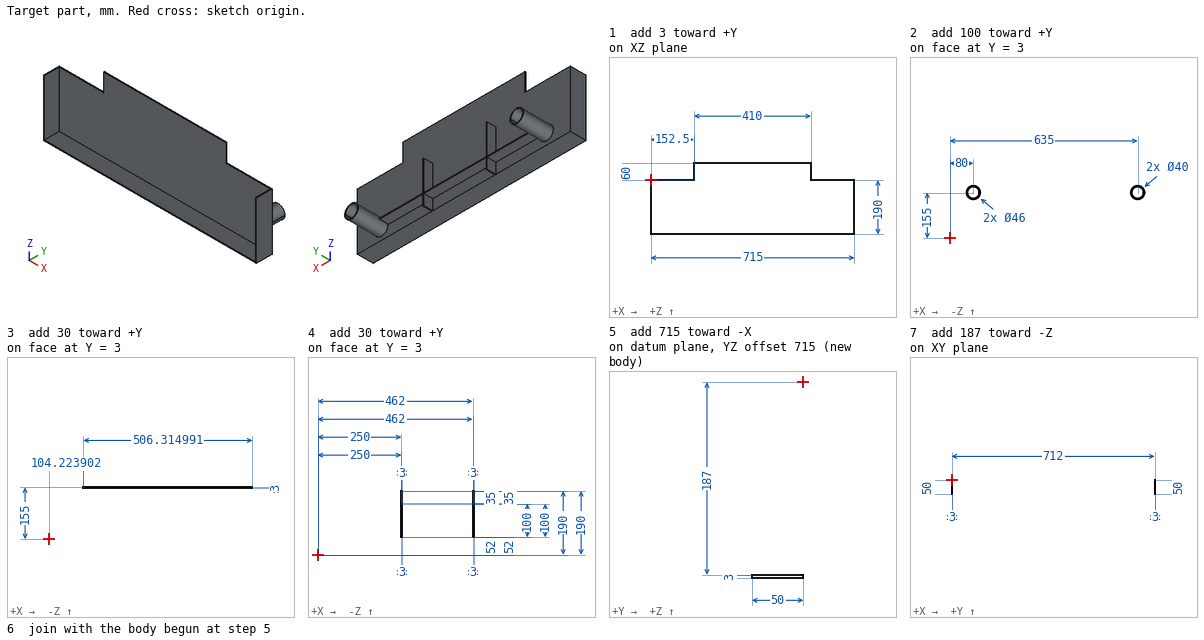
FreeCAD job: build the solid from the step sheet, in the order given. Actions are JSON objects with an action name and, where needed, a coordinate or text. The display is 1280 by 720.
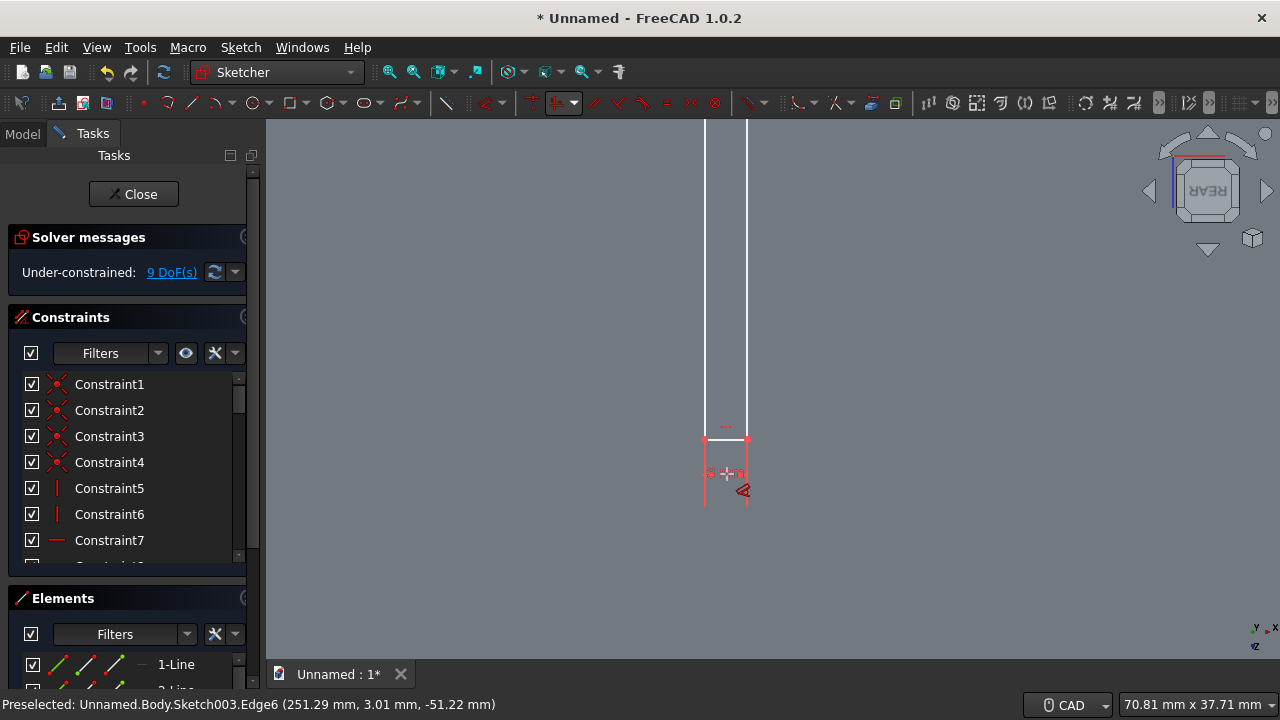
{"action": "scroll", "coordinate": [729, 446], "scroll_direction": "down", "scroll_amount": 12}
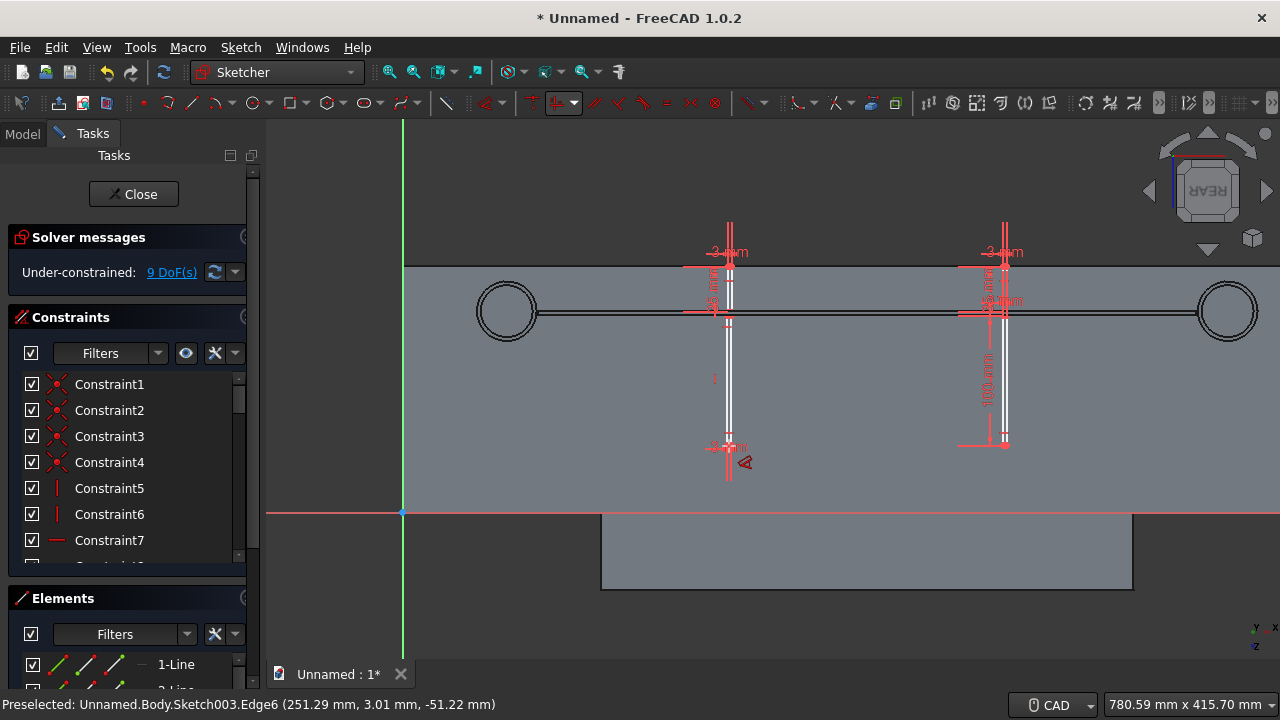
{"action": "scroll", "coordinate": [727, 420], "scroll_direction": "up", "scroll_amount": 7}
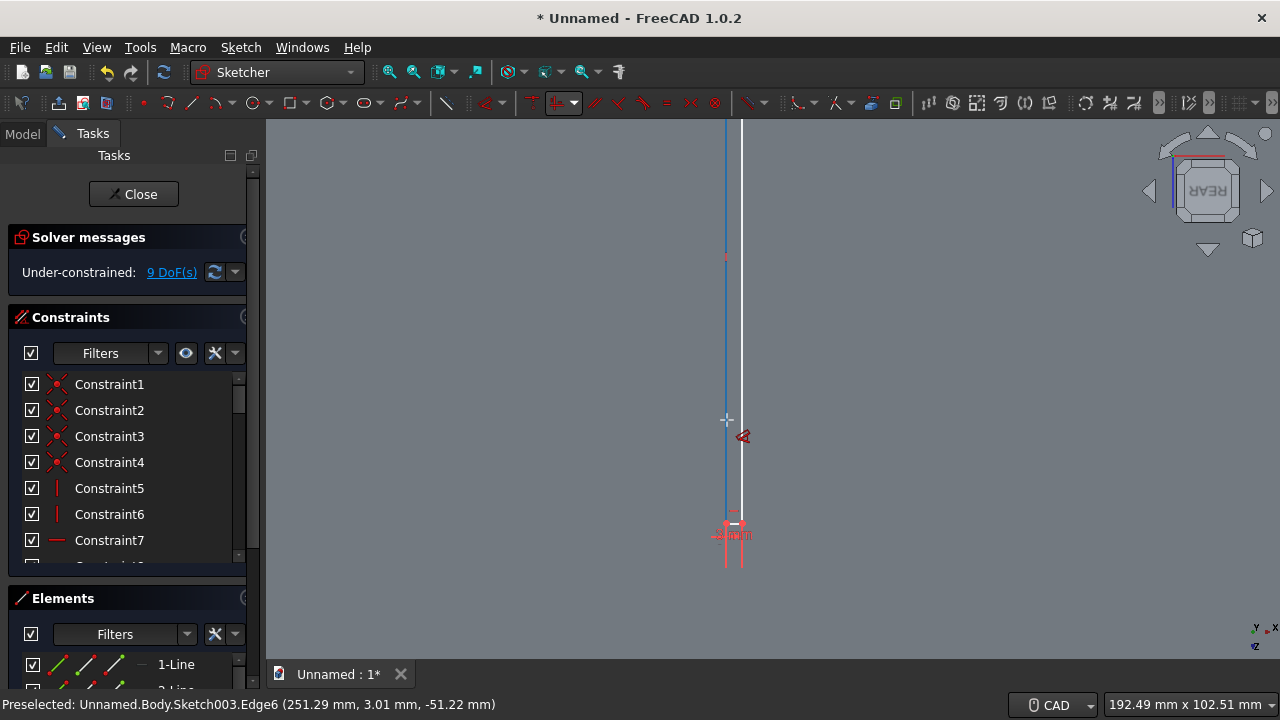
{"action": "left_click", "coordinate": [726, 418]}
{"action": "left_click", "coordinate": [760, 335]}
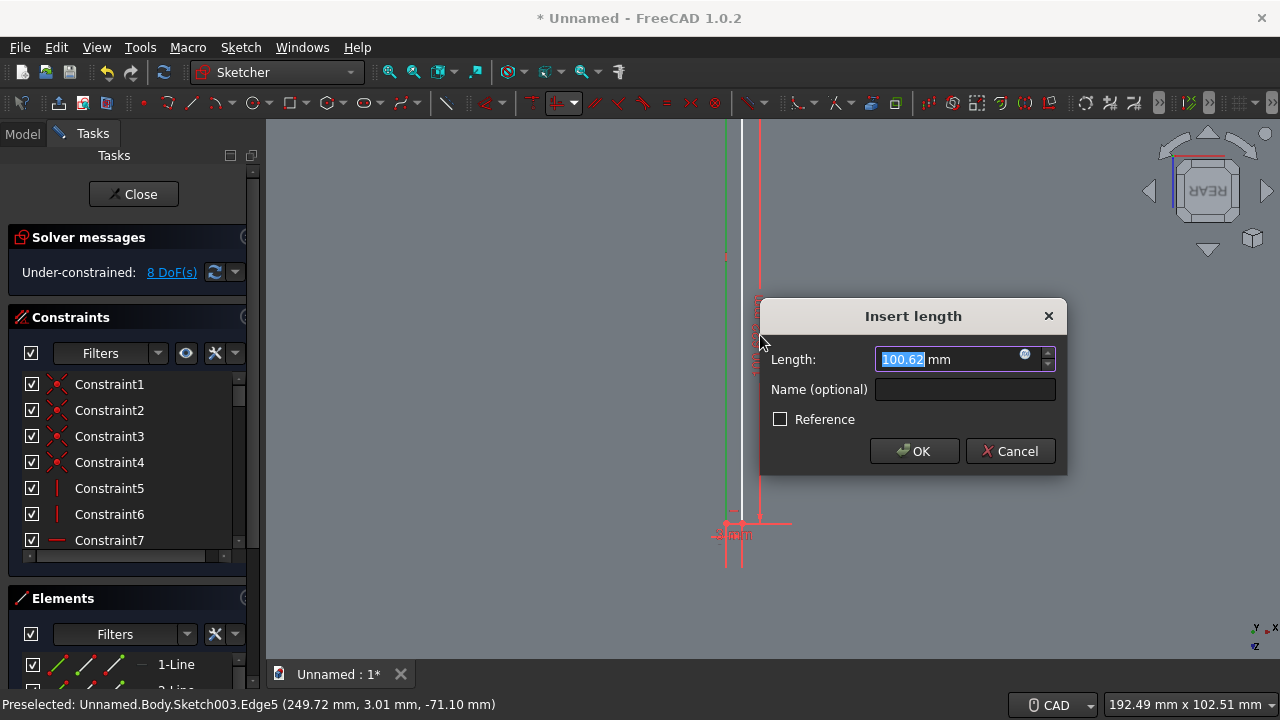
{"action": "type", "text": "100"}
{"action": "key", "text": "Return"}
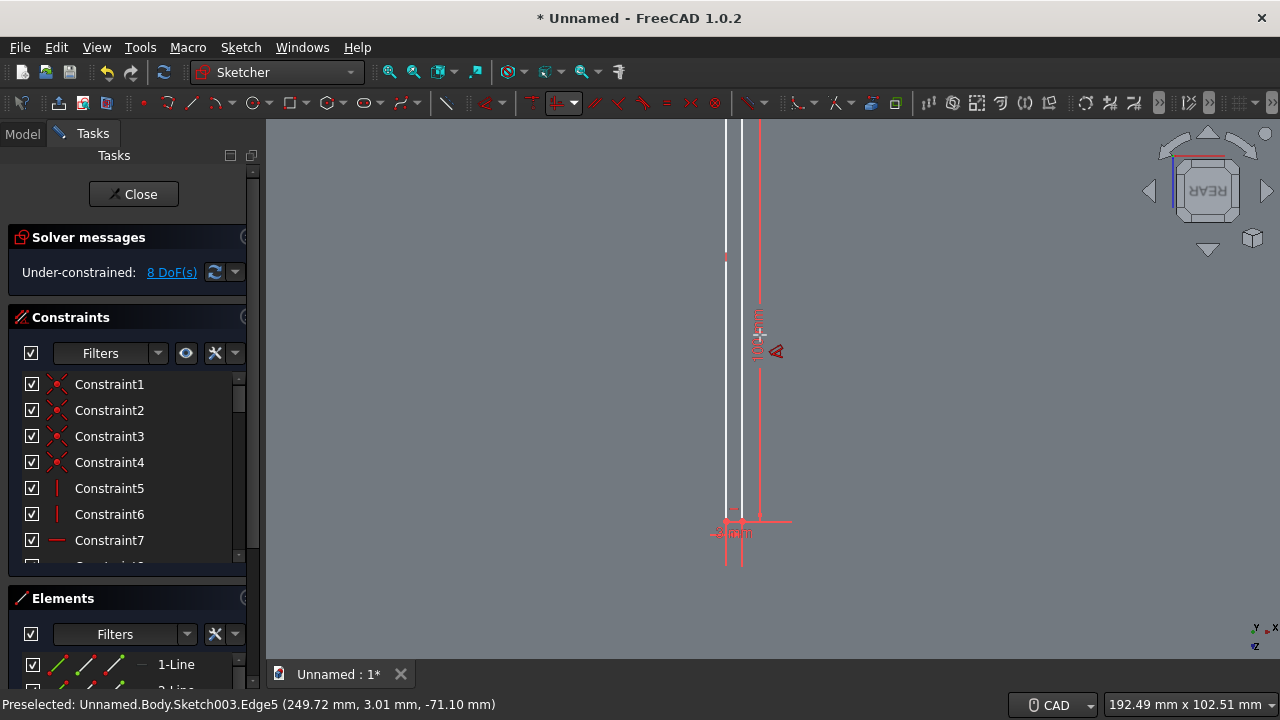
{"action": "left_click", "coordinate": [726, 522]}
{"action": "left_click", "coordinate": [760, 576]}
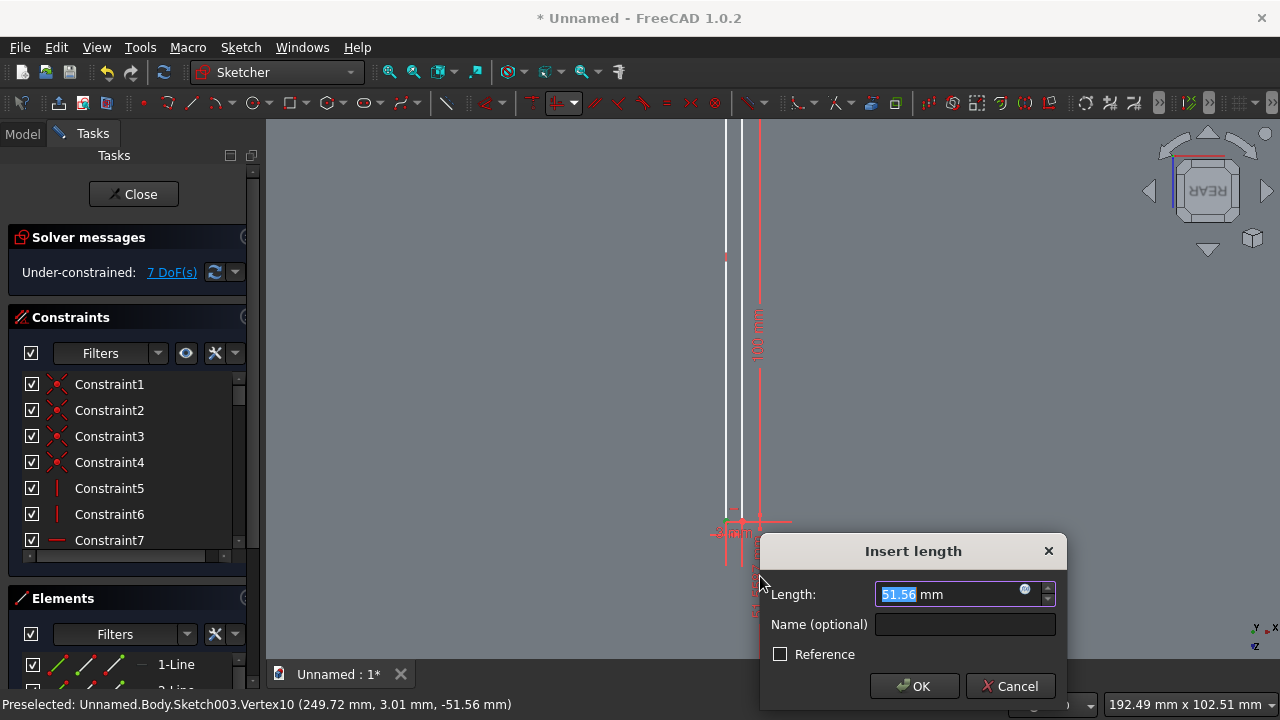
{"action": "type", "text": "52"}
{"action": "key", "text": "Return"}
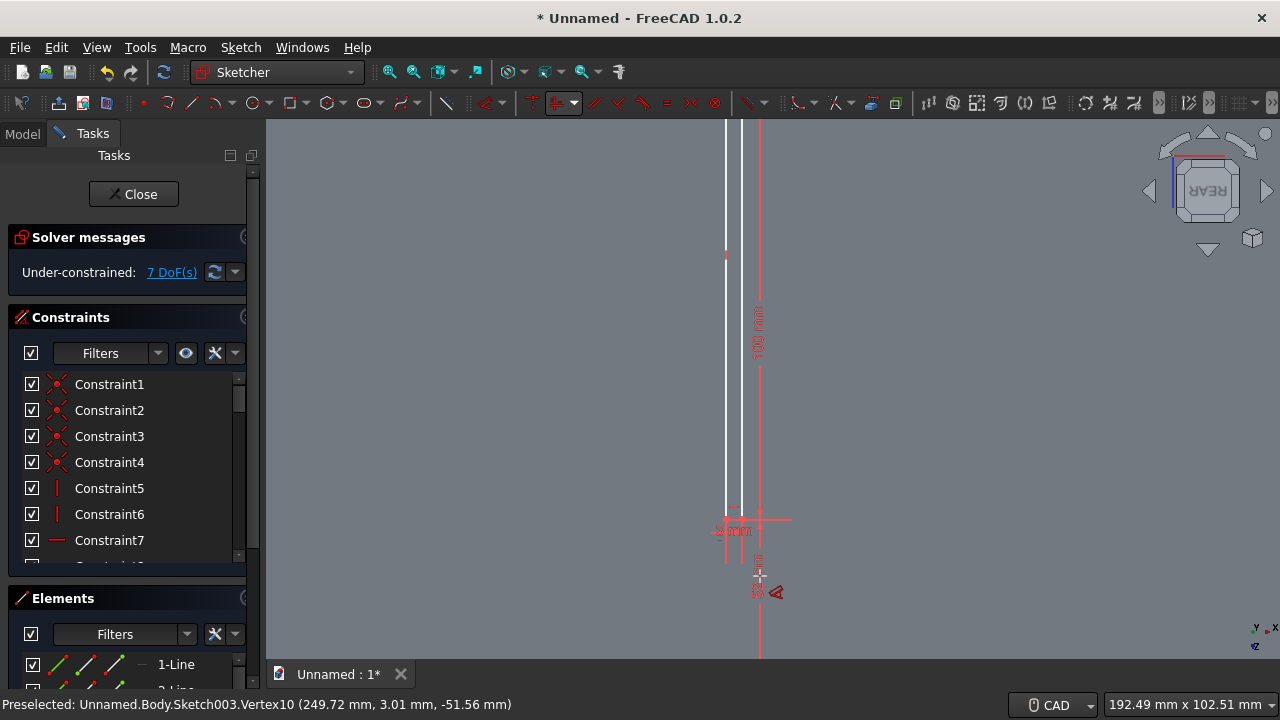
{"action": "scroll", "coordinate": [727, 420], "scroll_direction": "down", "scroll_amount": 7}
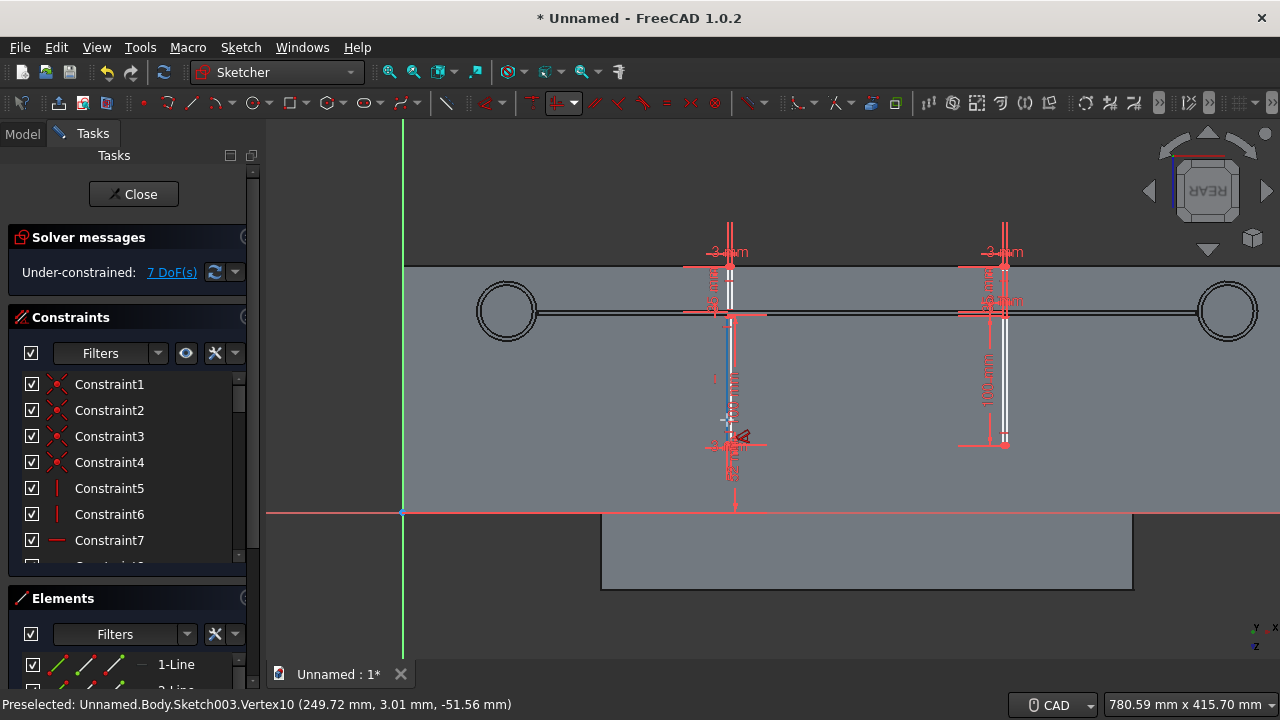
{"action": "scroll", "coordinate": [1003, 446], "scroll_direction": "up", "scroll_amount": 6}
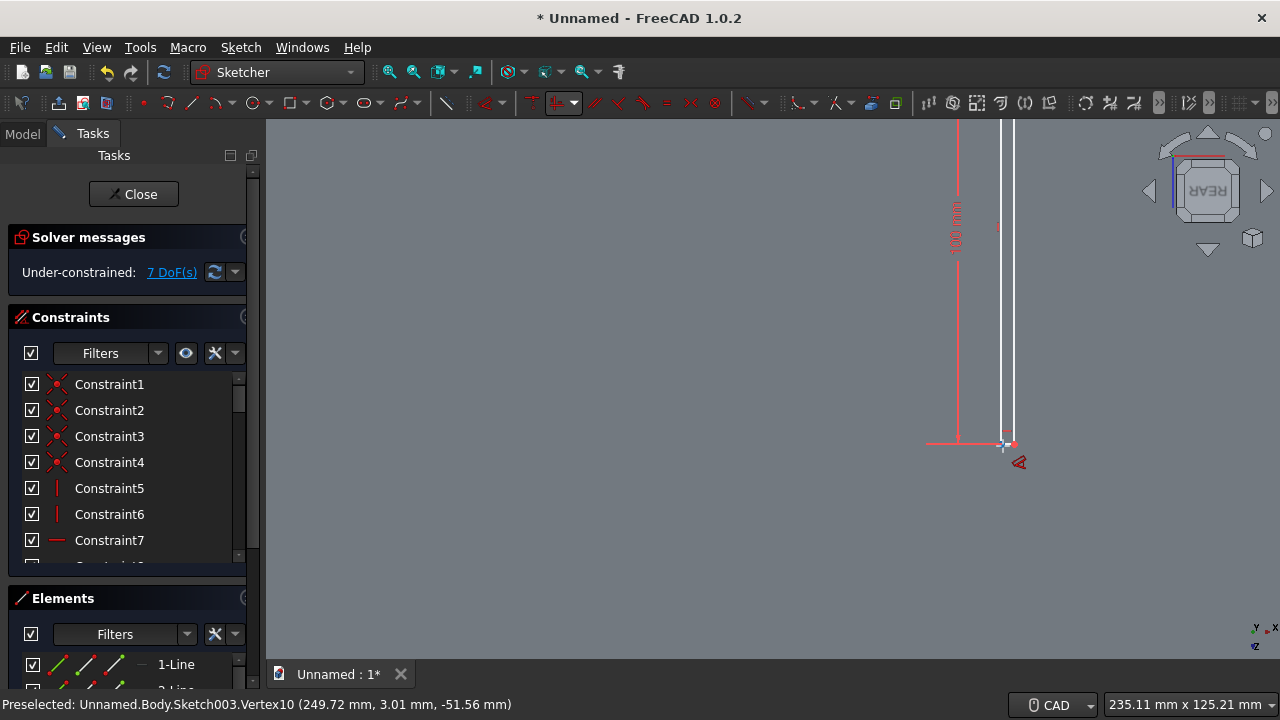
{"action": "left_click", "coordinate": [1001, 444]}
{"action": "left_click", "coordinate": [1035, 538]}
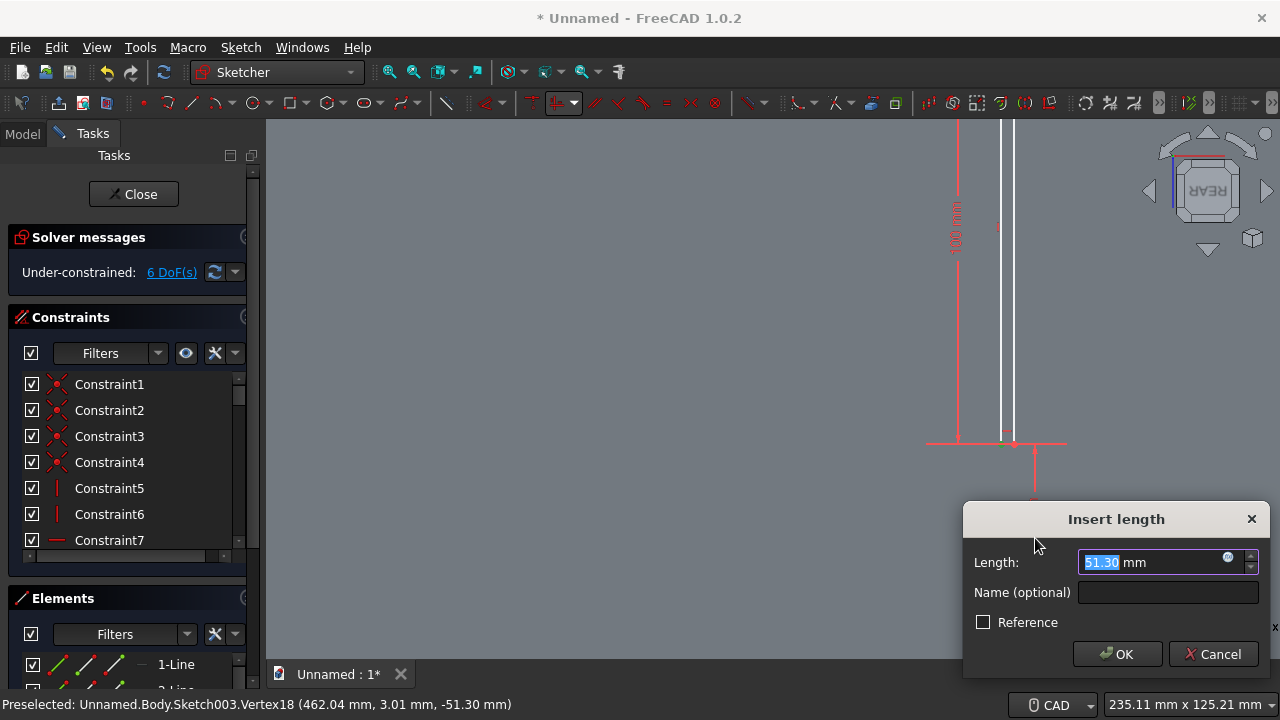
{"action": "type", "text": "52"}
{"action": "key", "text": "Return"}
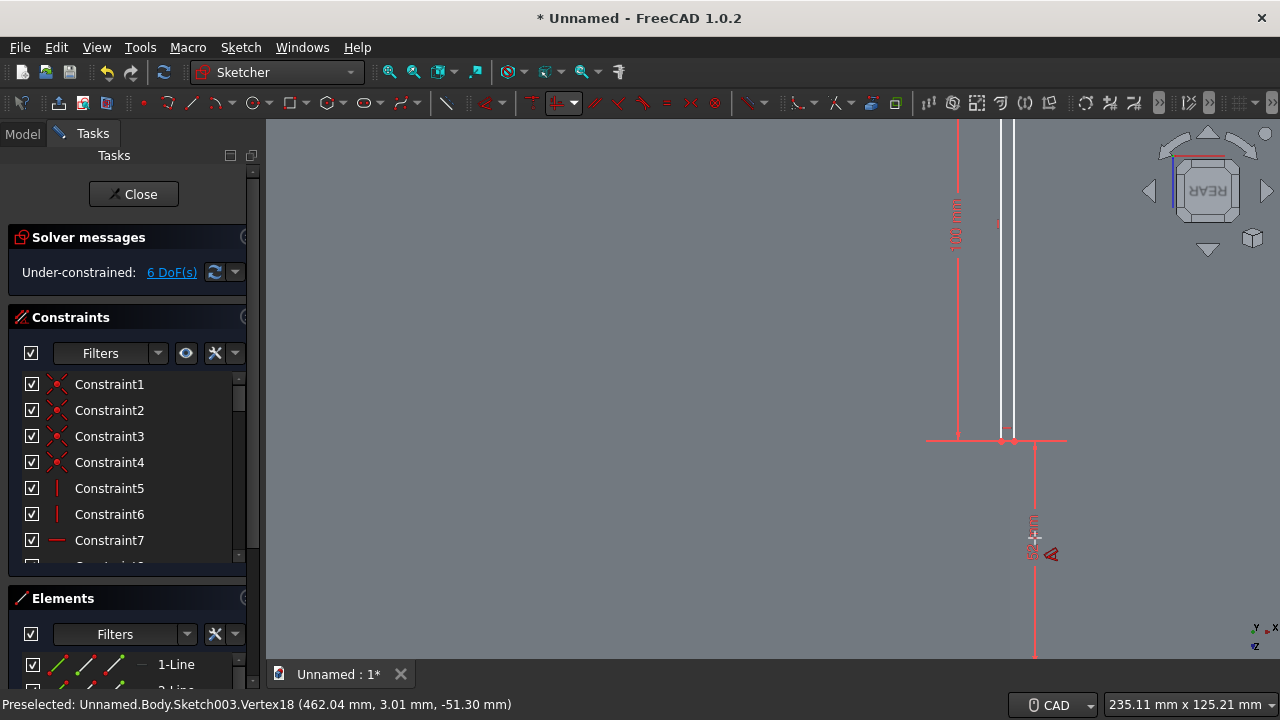
{"action": "scroll", "coordinate": [1003, 446], "scroll_direction": "down", "scroll_amount": 6}